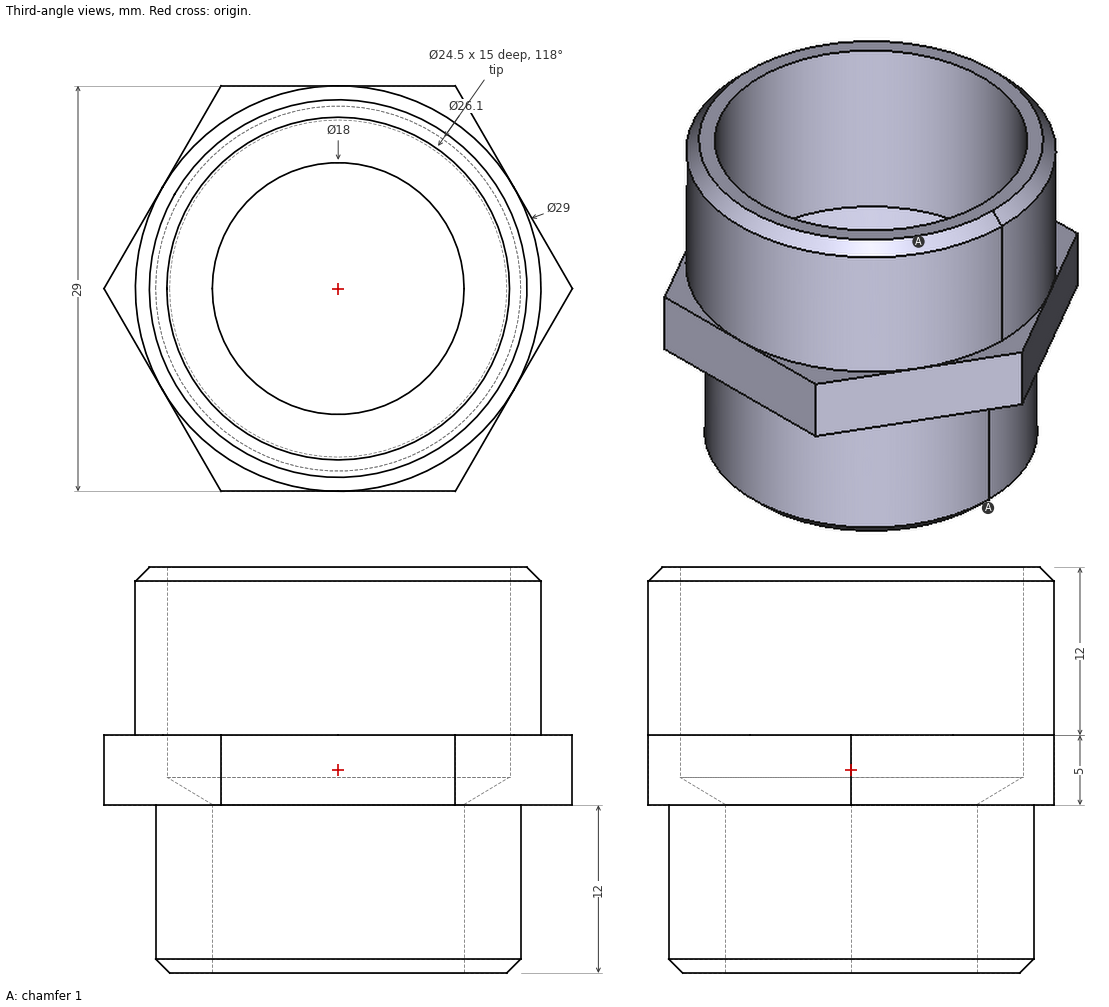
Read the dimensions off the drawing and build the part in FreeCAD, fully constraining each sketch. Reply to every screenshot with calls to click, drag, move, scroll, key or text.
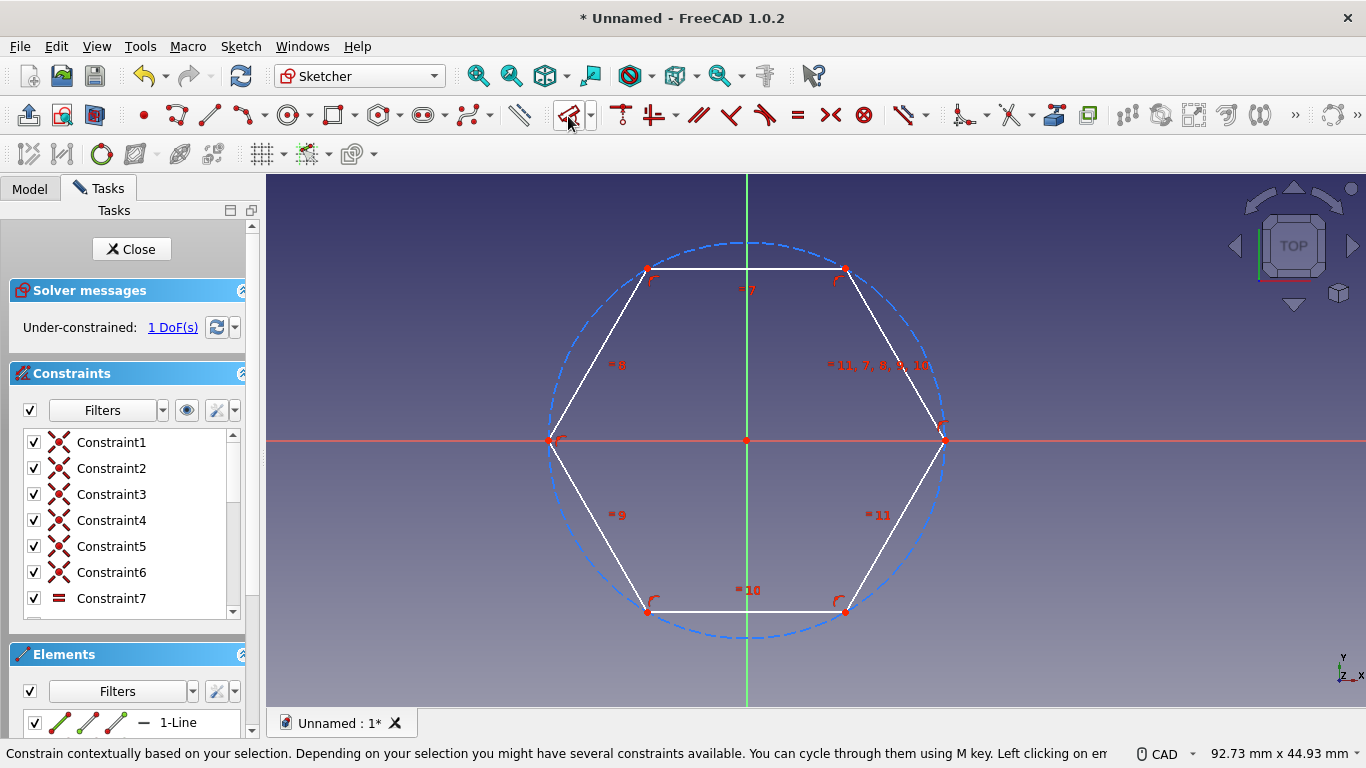
click(648, 612)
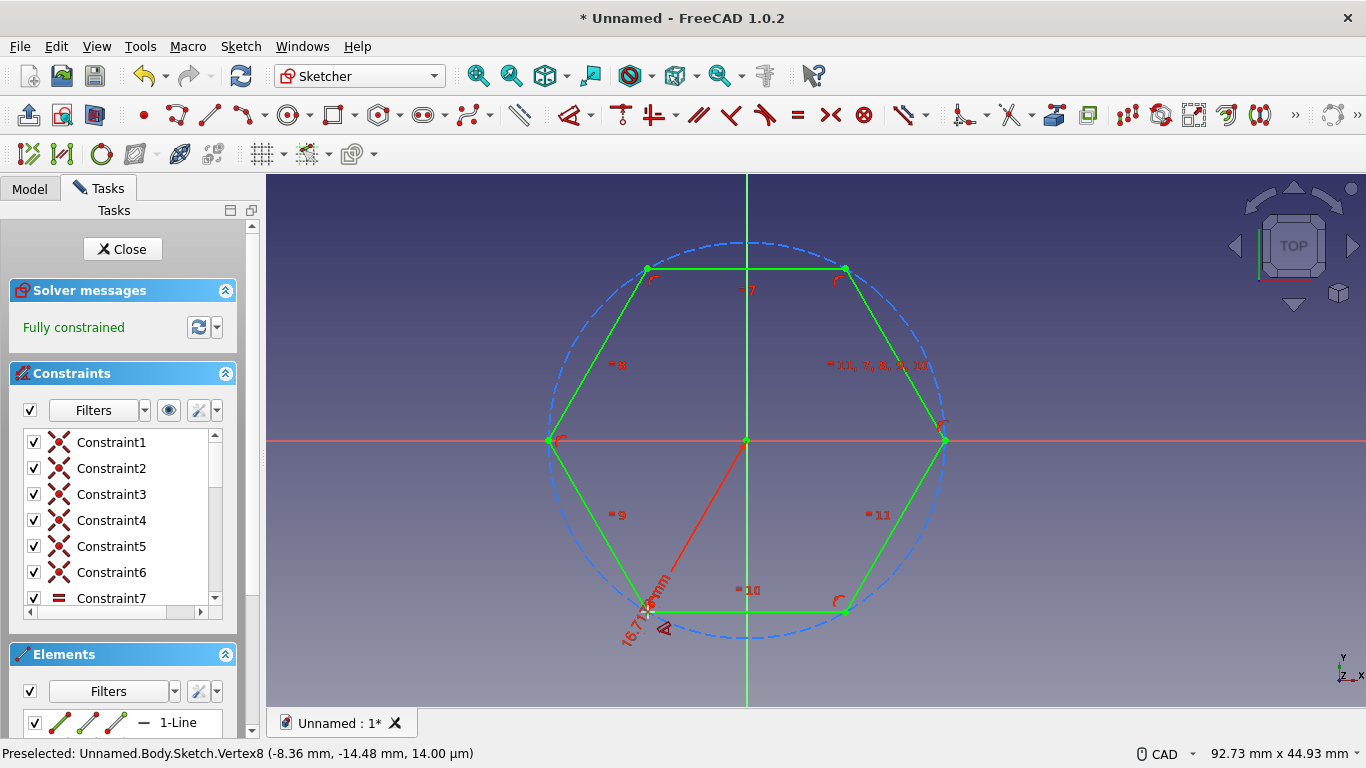
click(846, 269)
click(880, 362)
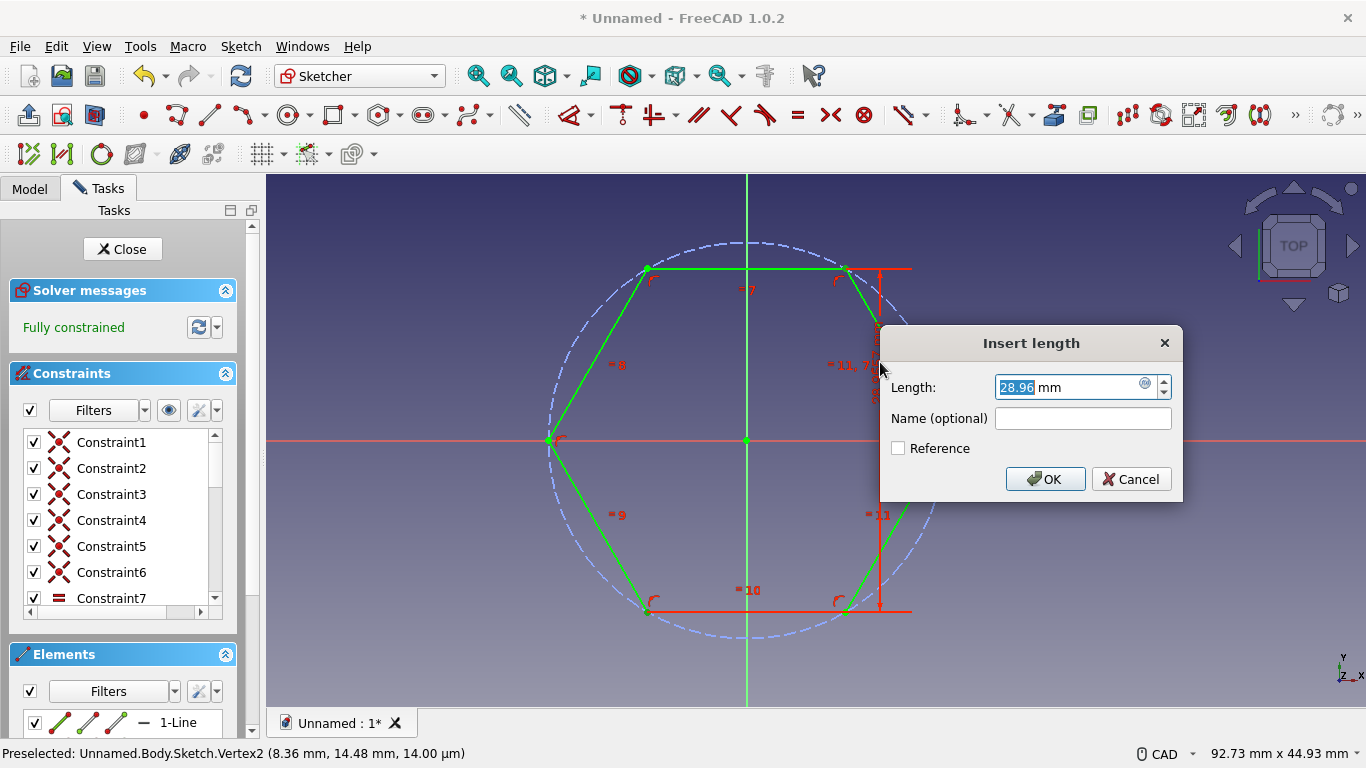
text(29)
key(Return)
key(Escape)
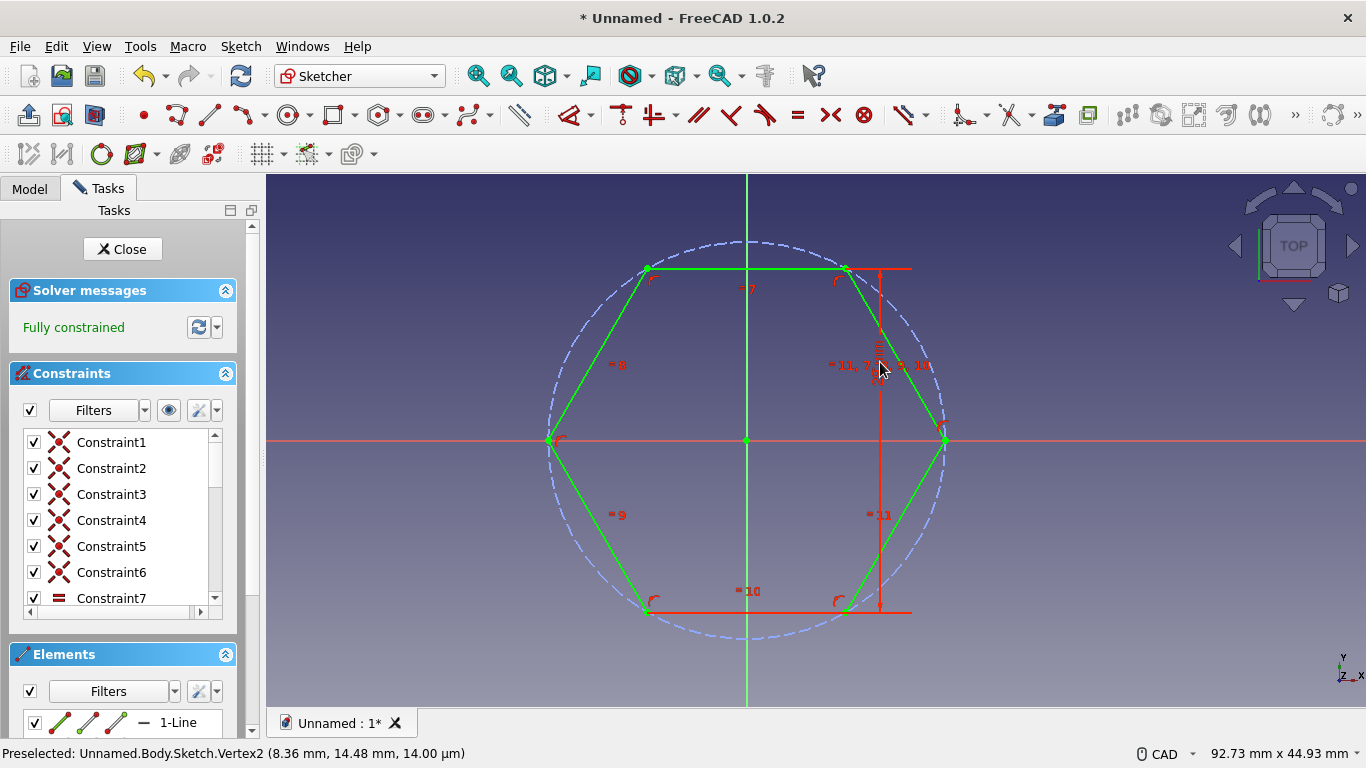
click(123, 249)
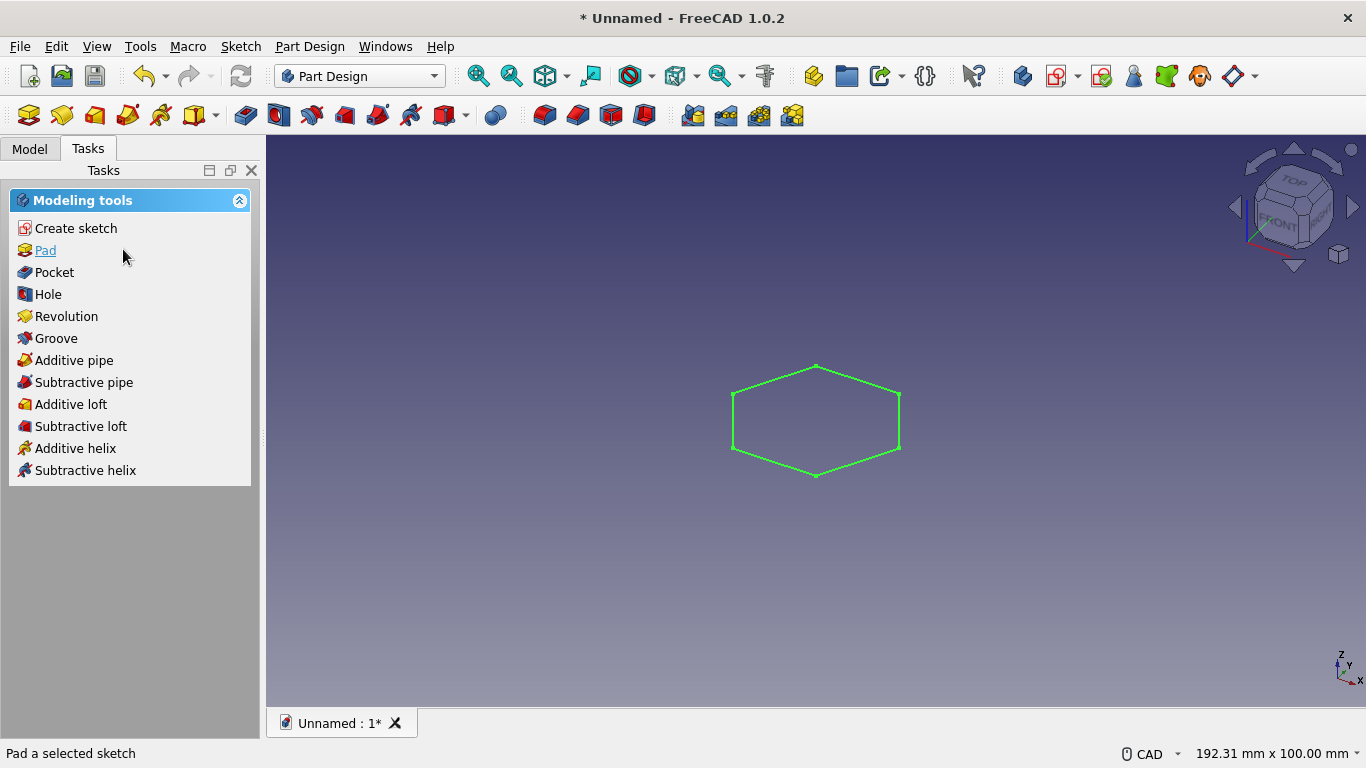
click(29, 116)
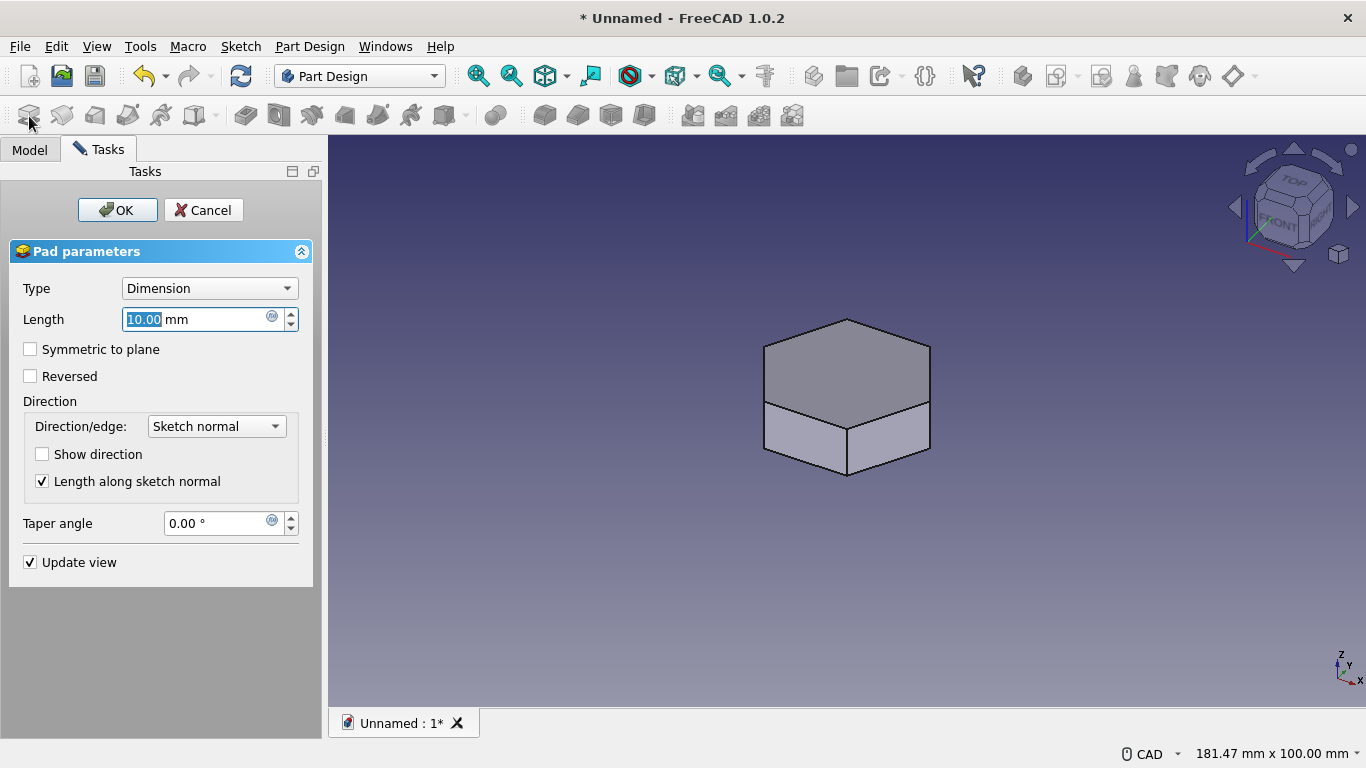
text(5)
key(Tab)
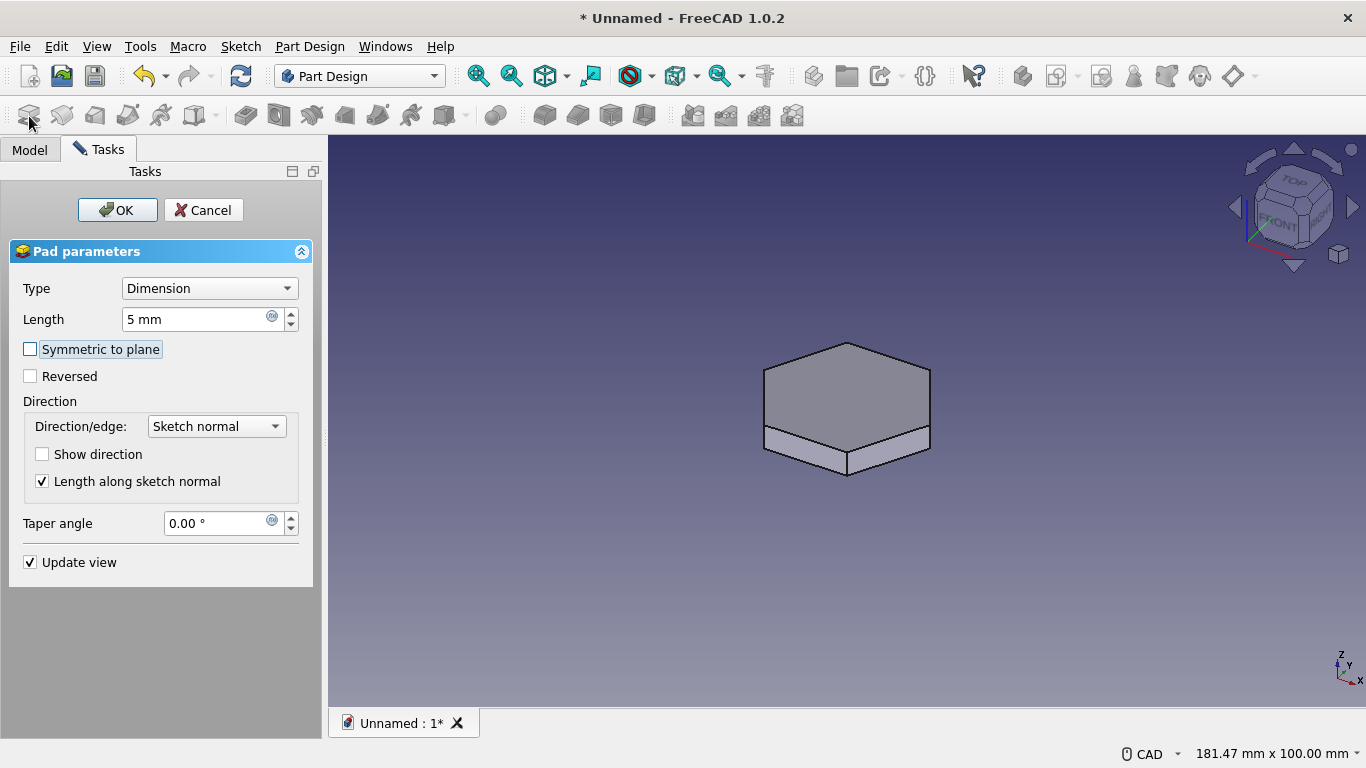
click(31, 349)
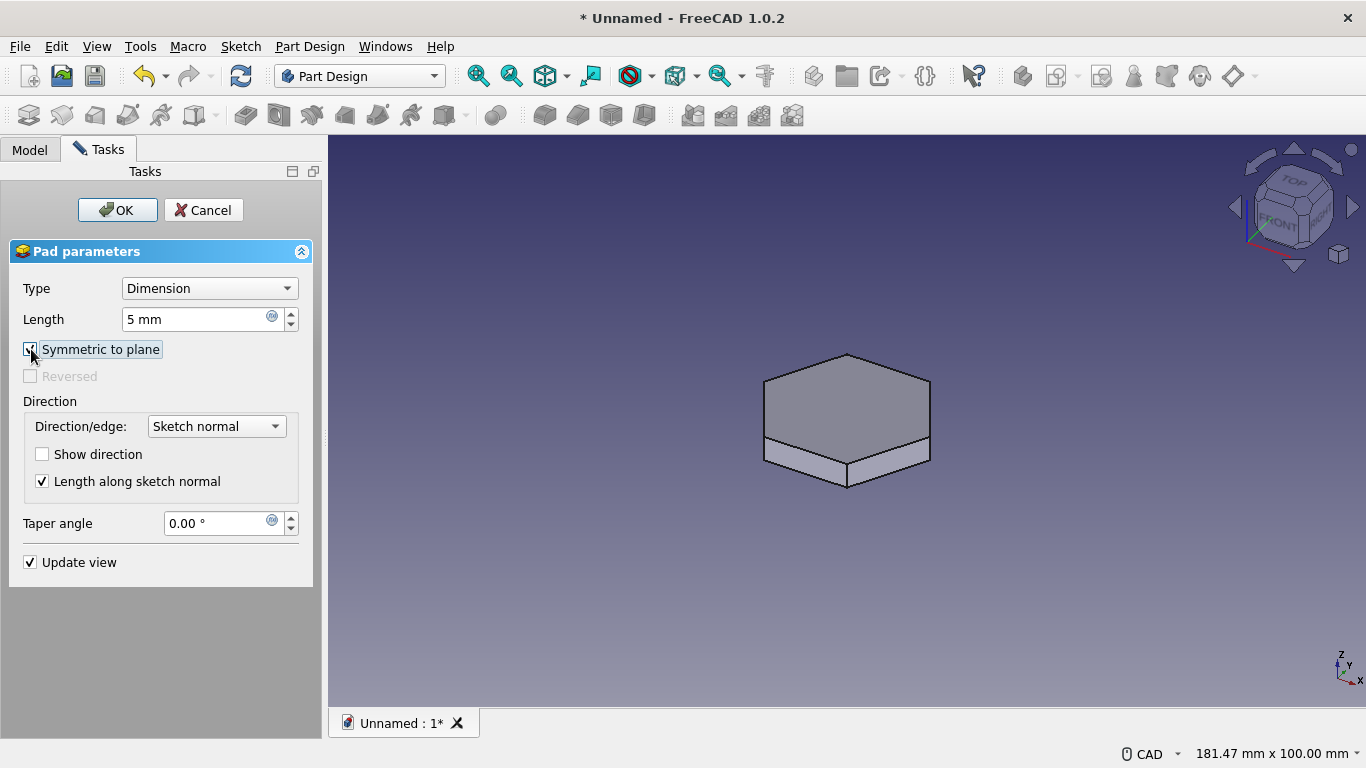
click(118, 210)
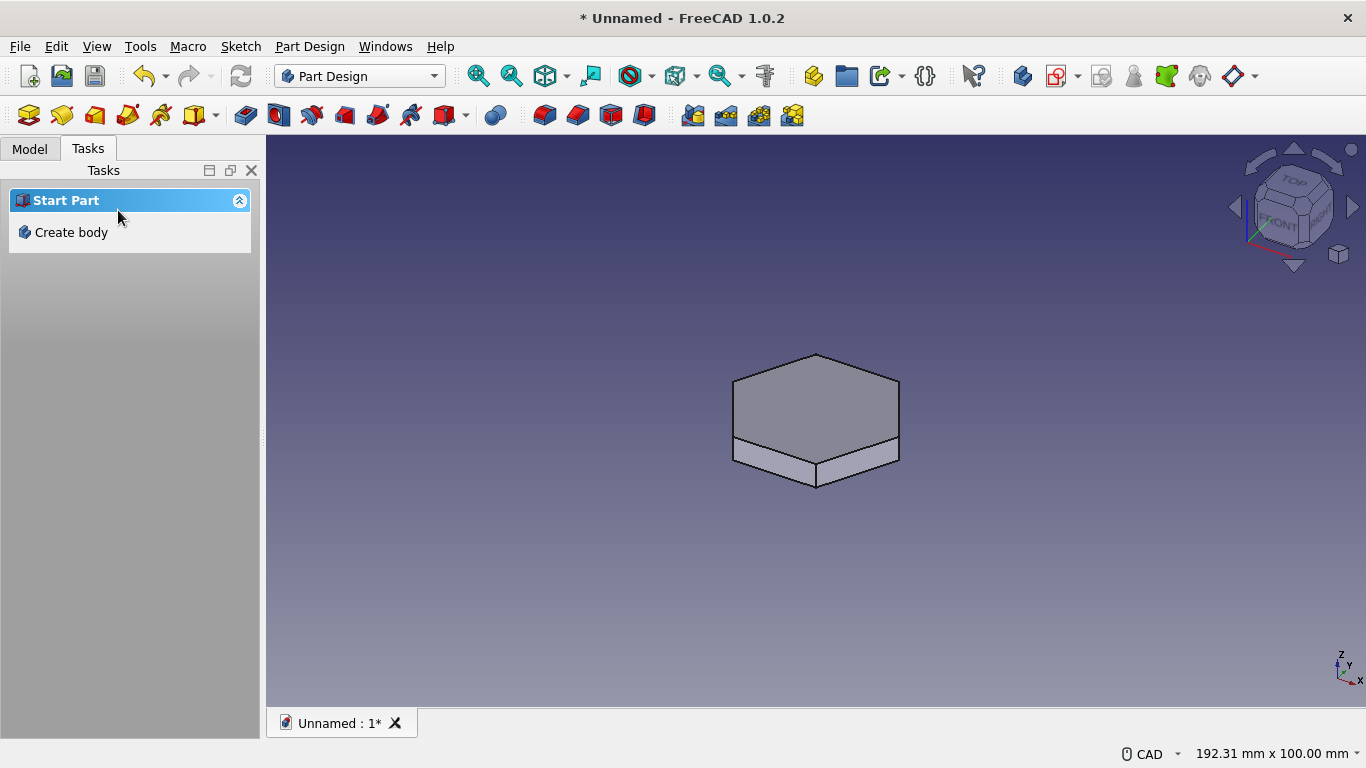
click(479, 76)